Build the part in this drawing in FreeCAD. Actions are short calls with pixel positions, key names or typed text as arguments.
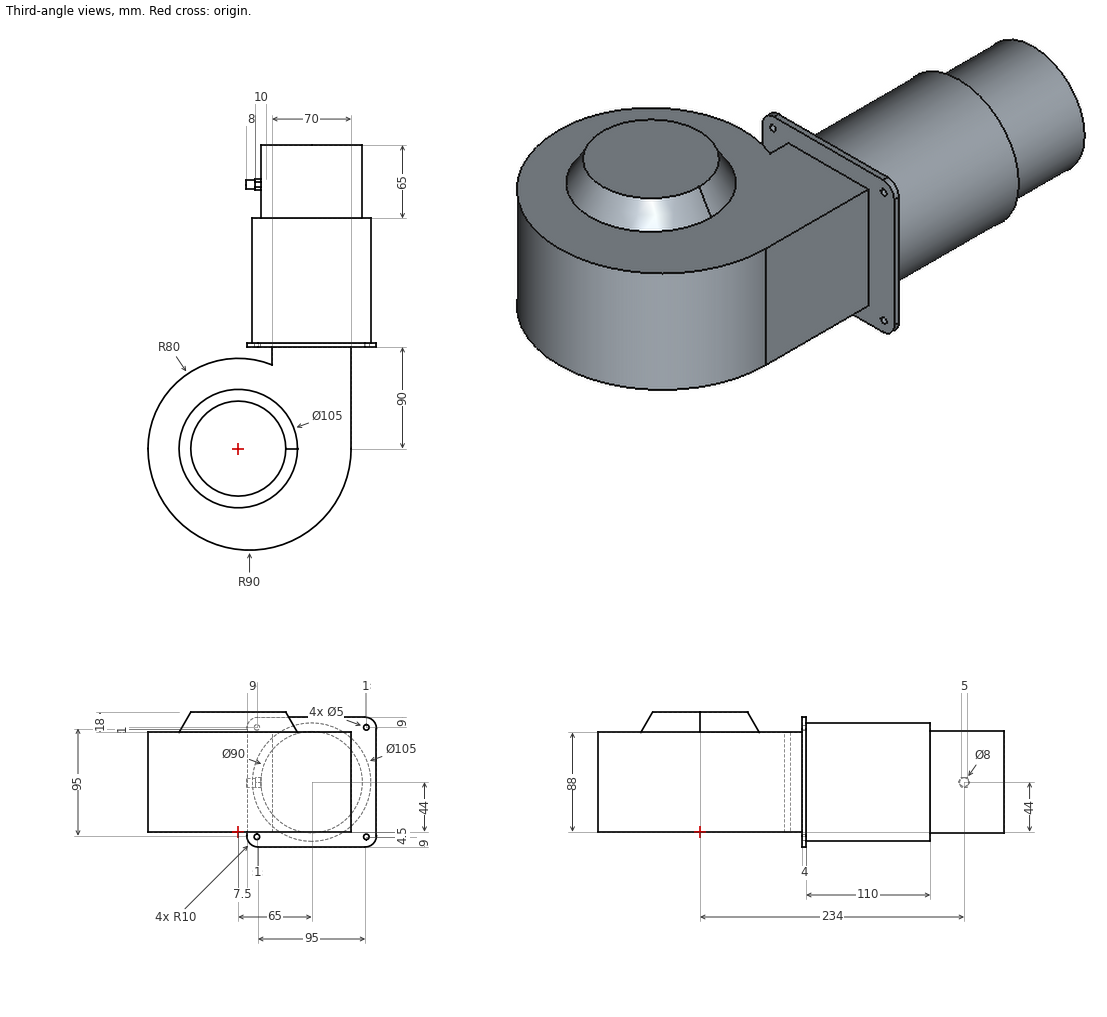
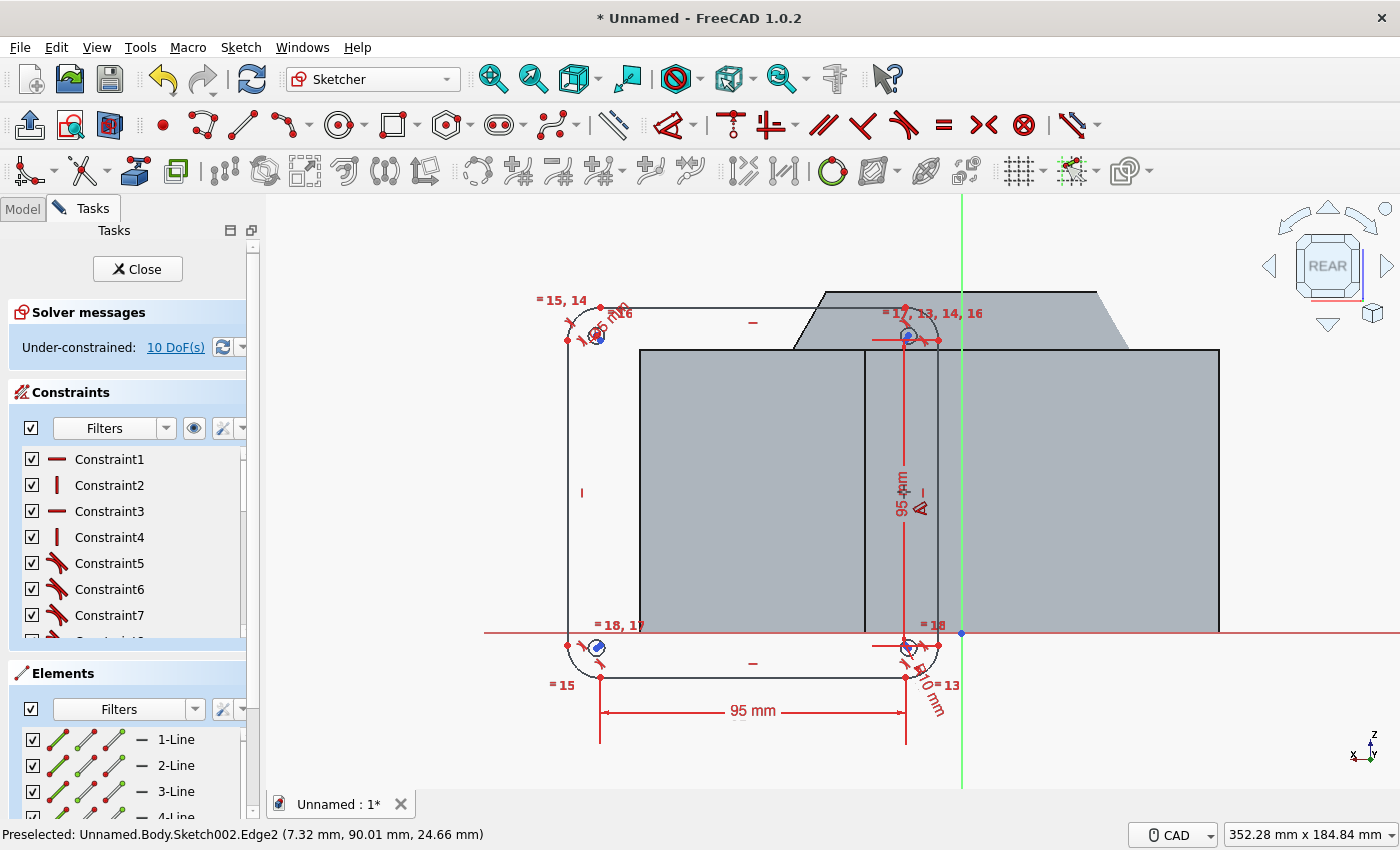
scroll(600, 308, up, 13)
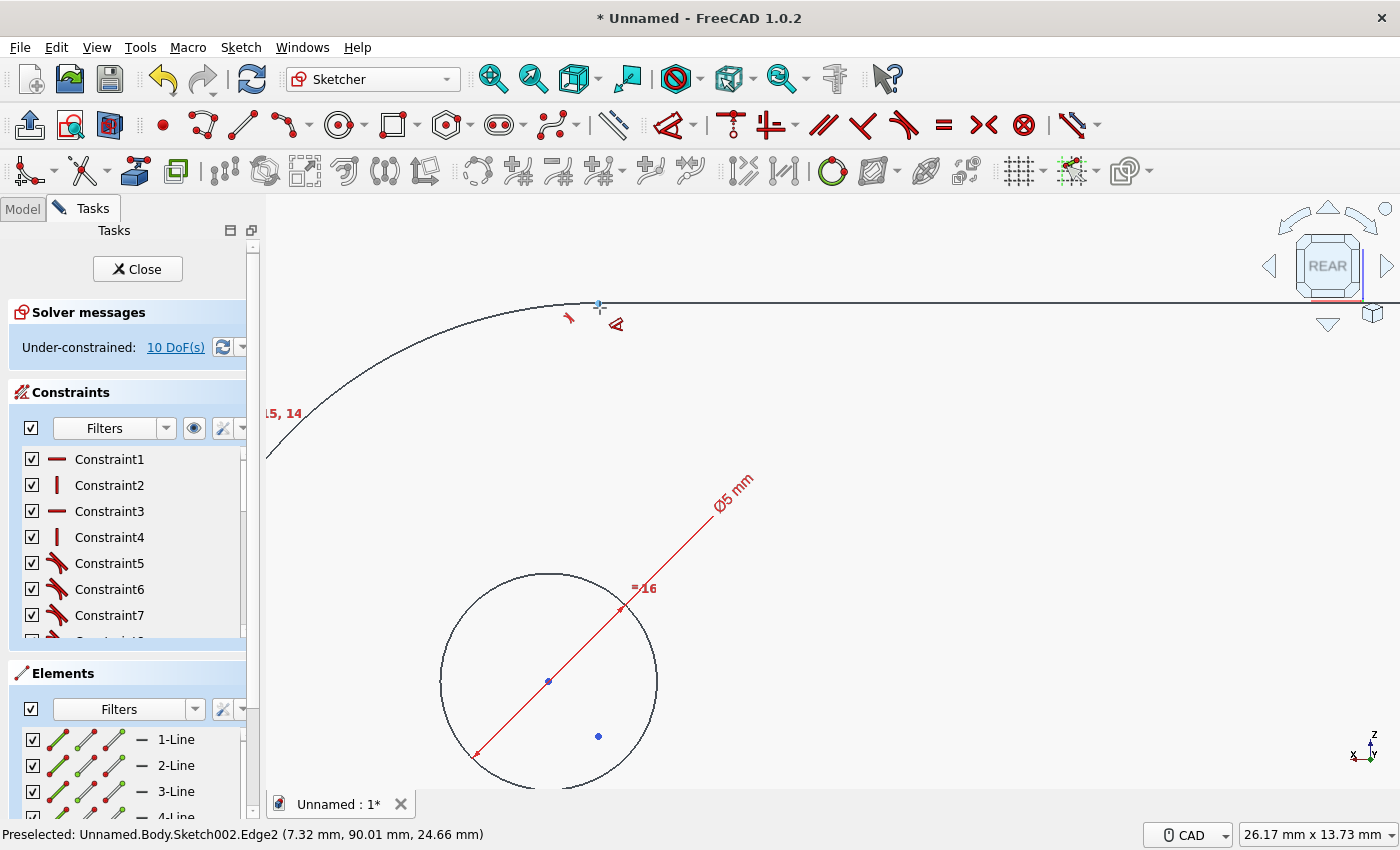
click(599, 303)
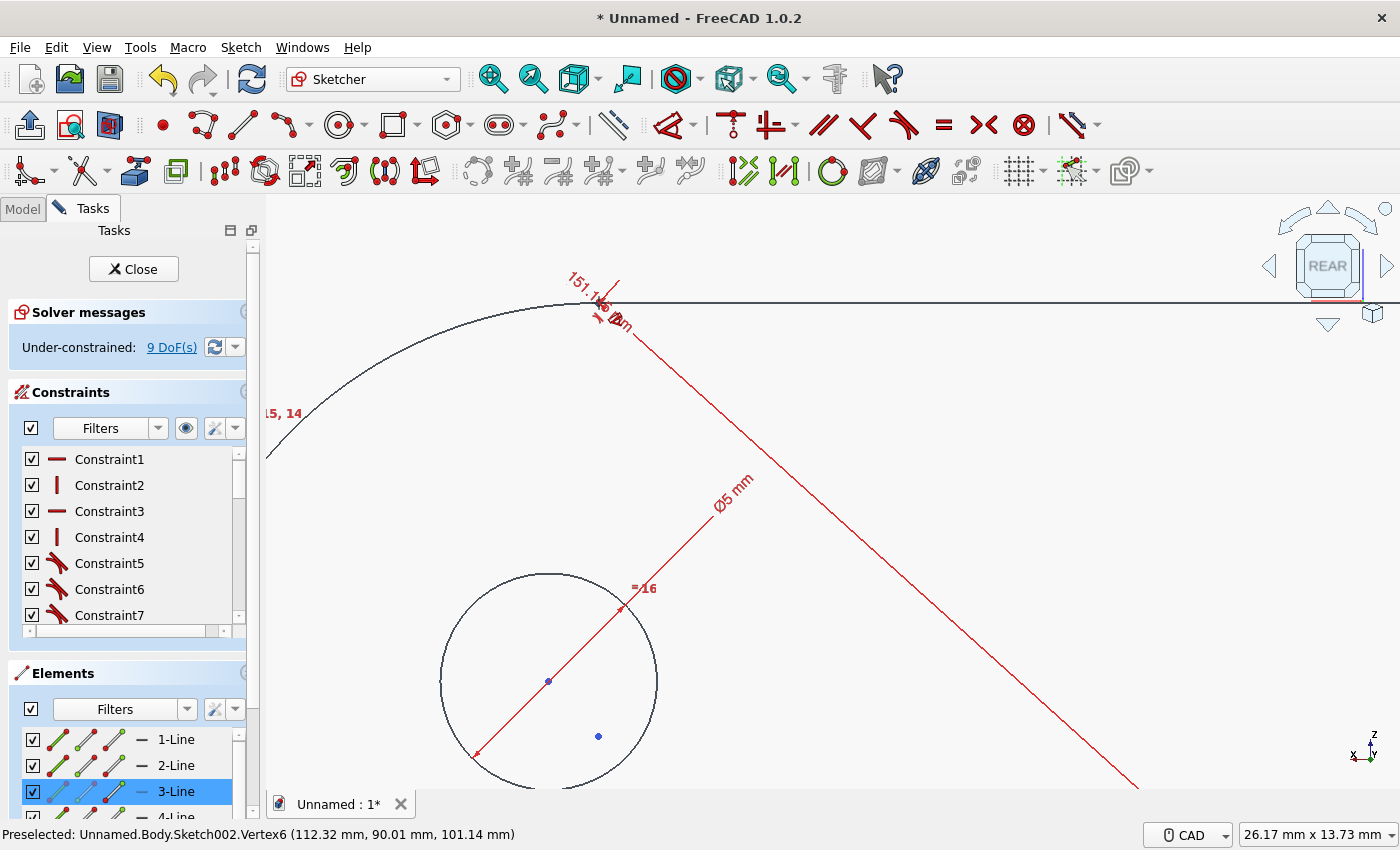
click(549, 682)
click(574, 269)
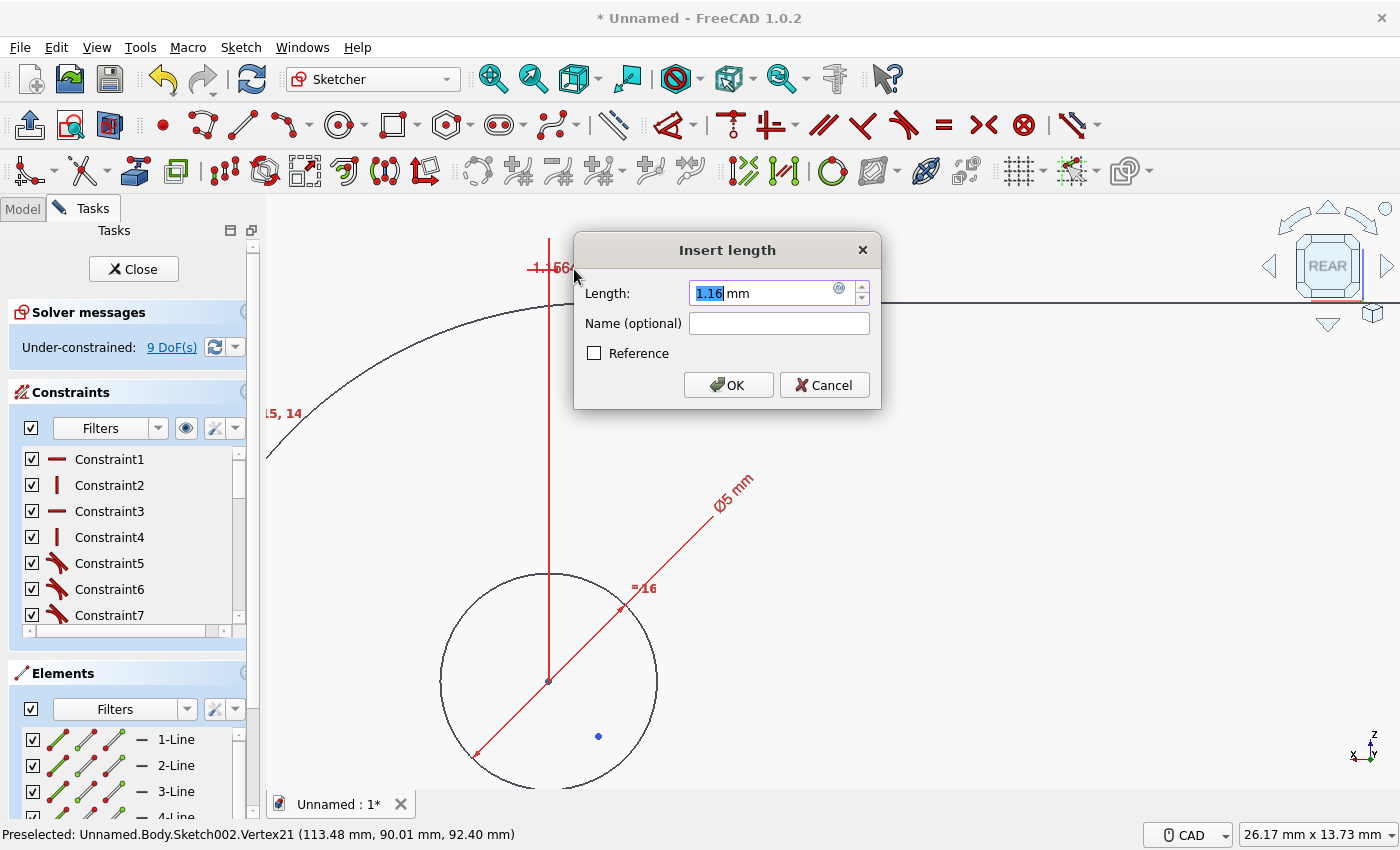
text(1)
key(Return)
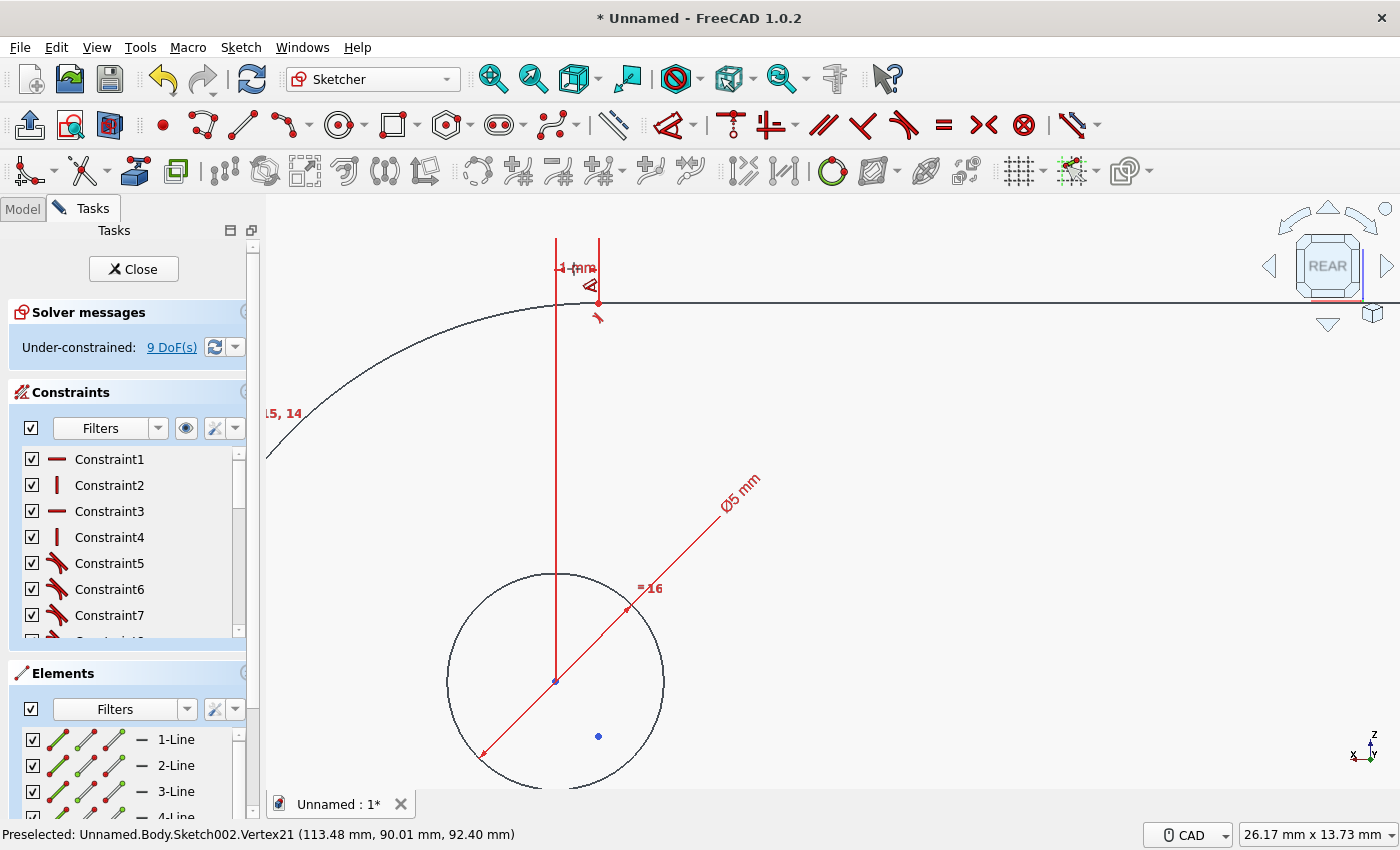
scroll(600, 308, down, 13)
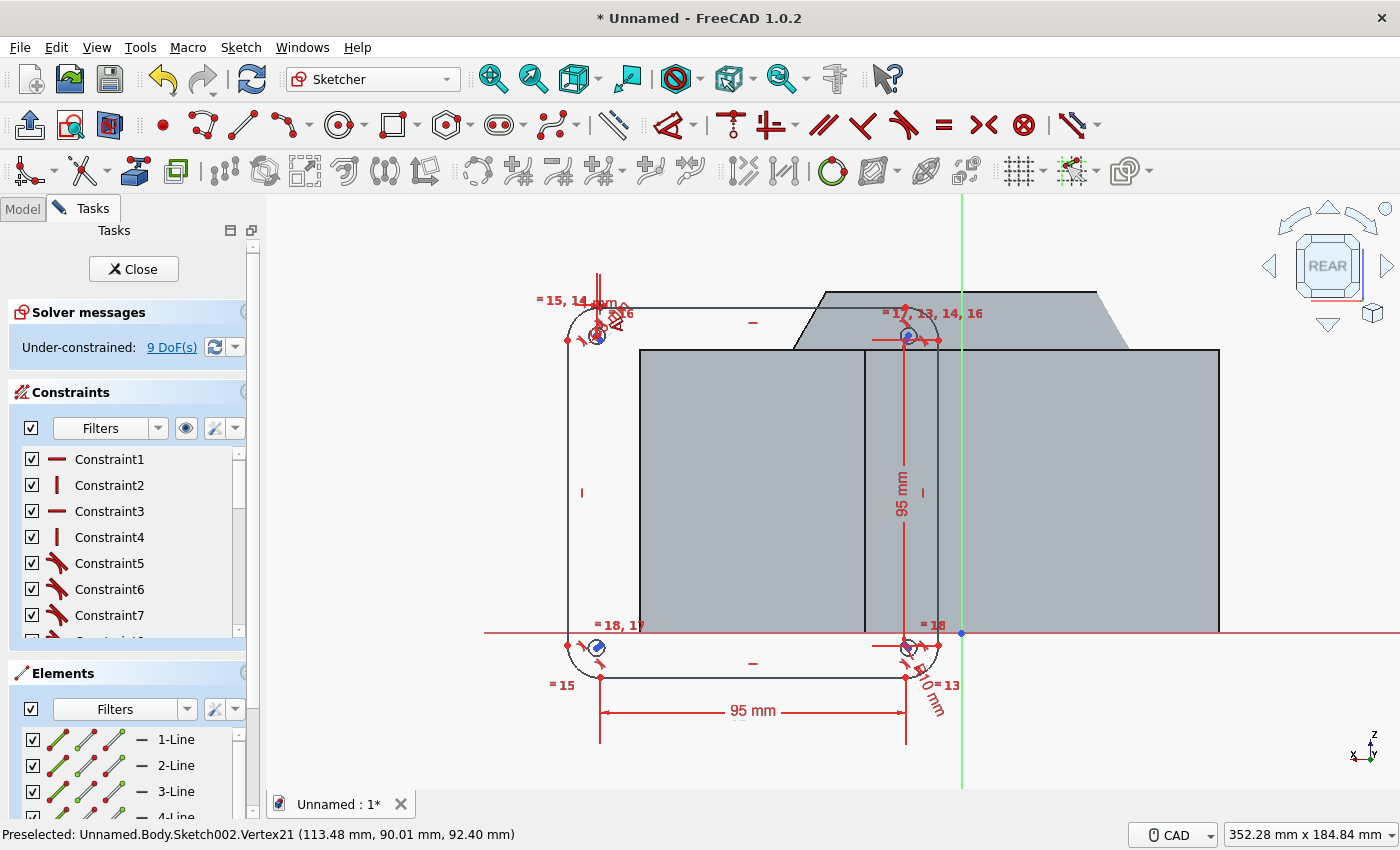
scroll(600, 308, up, 2)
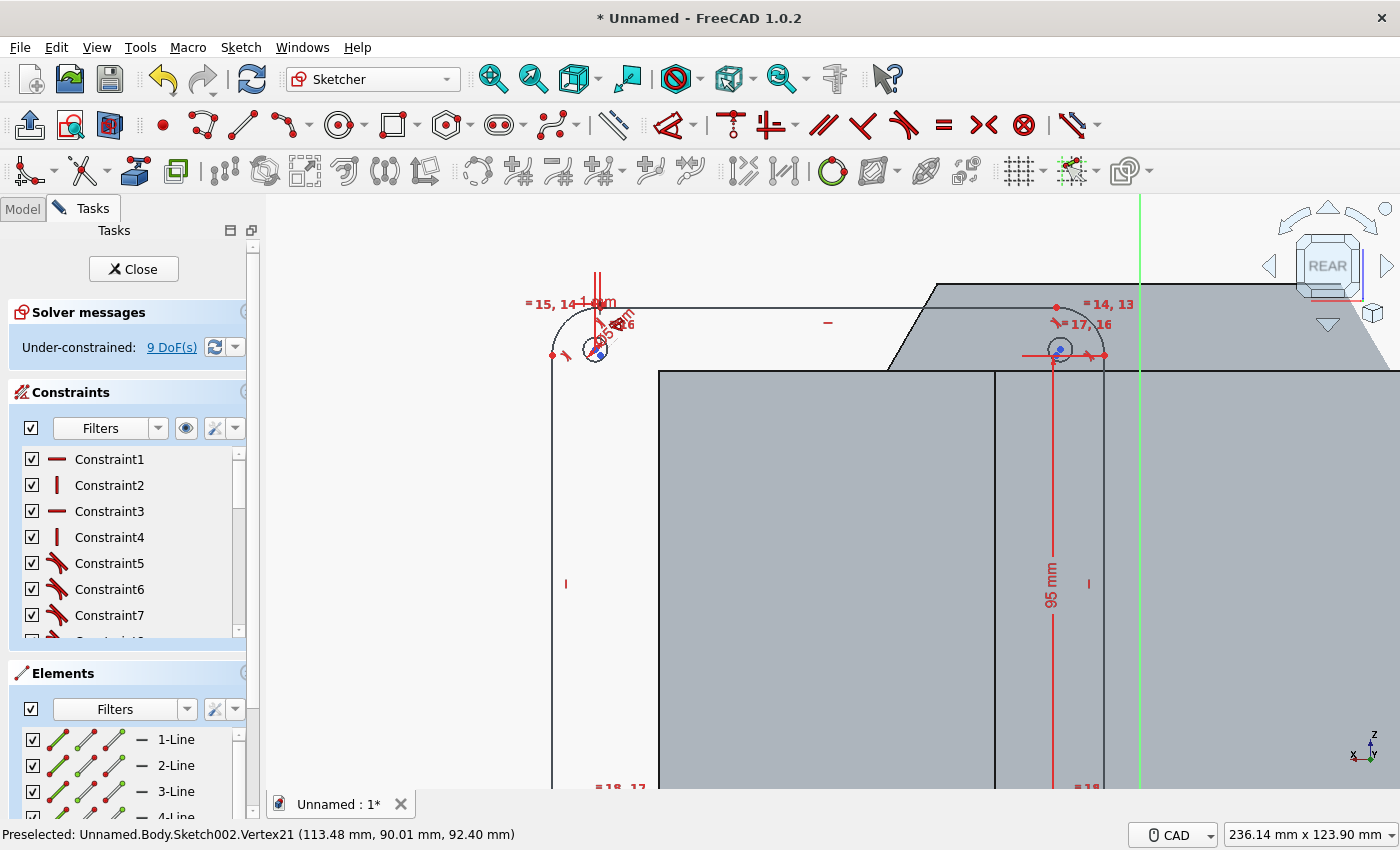
click(600, 308)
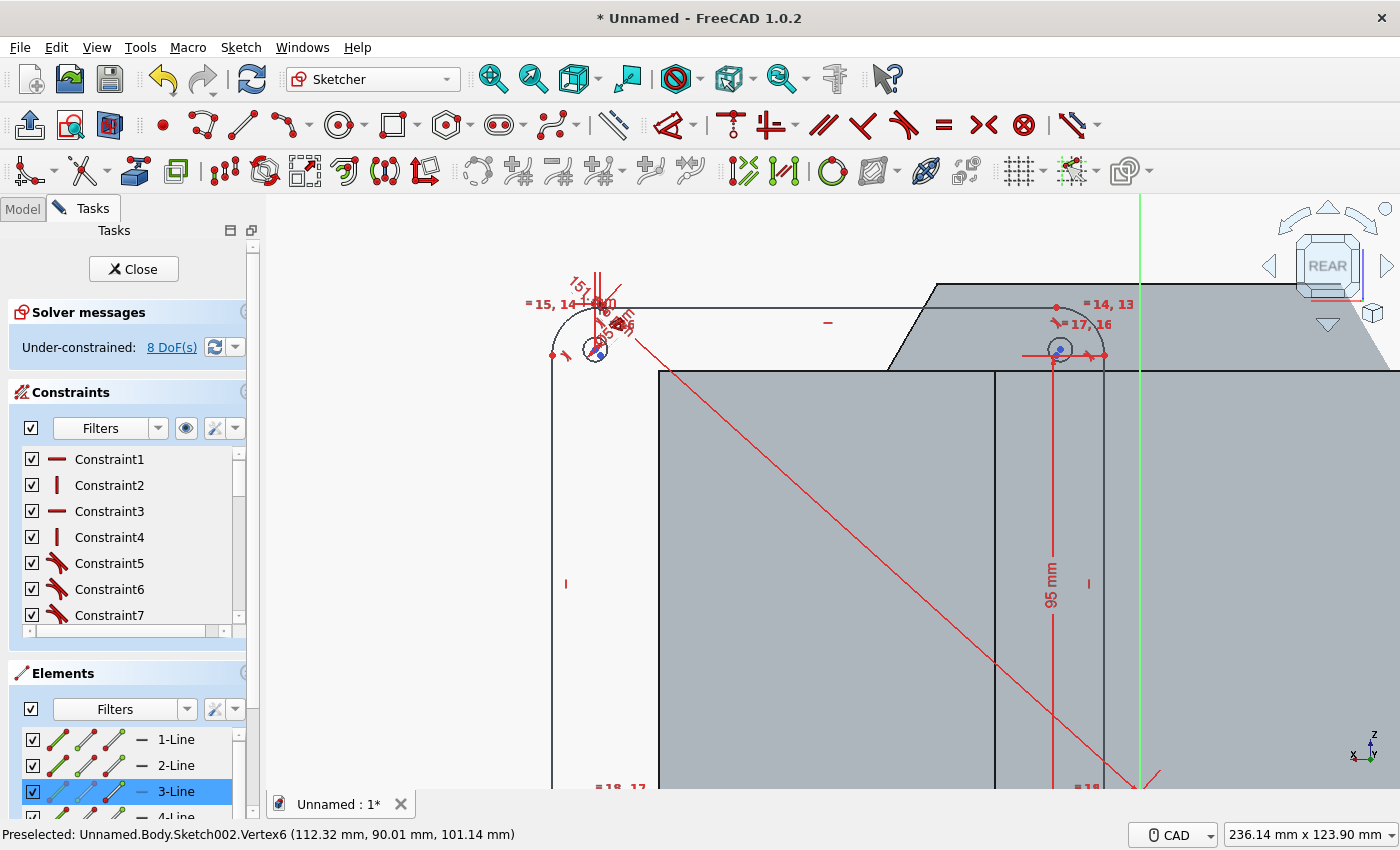
scroll(595, 350, up, 3)